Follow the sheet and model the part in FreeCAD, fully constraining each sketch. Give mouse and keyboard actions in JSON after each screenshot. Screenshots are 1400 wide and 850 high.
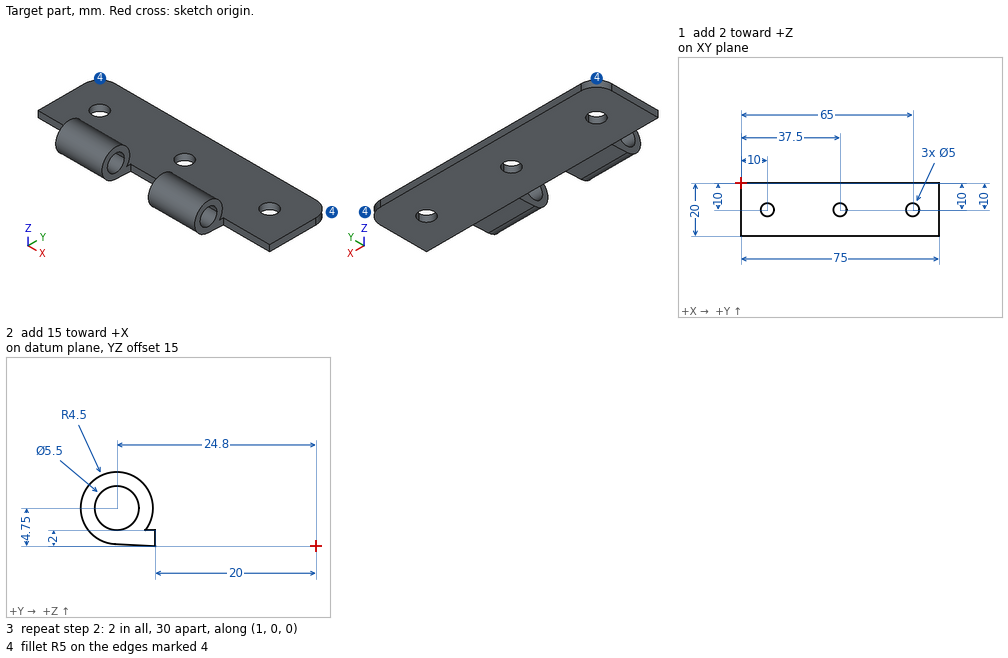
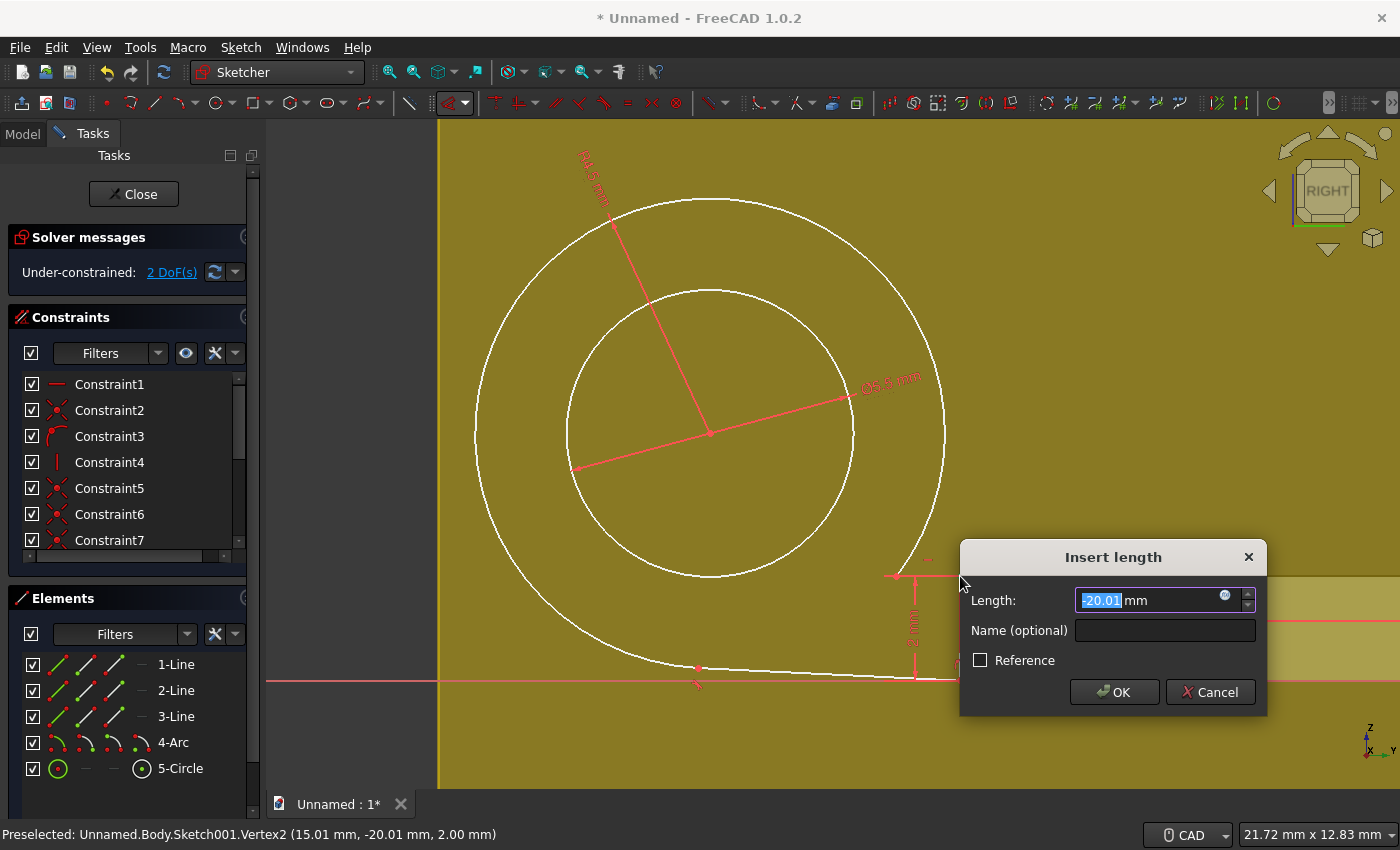
{"action": "type", "text": "-20"}
{"action": "key", "text": "Return"}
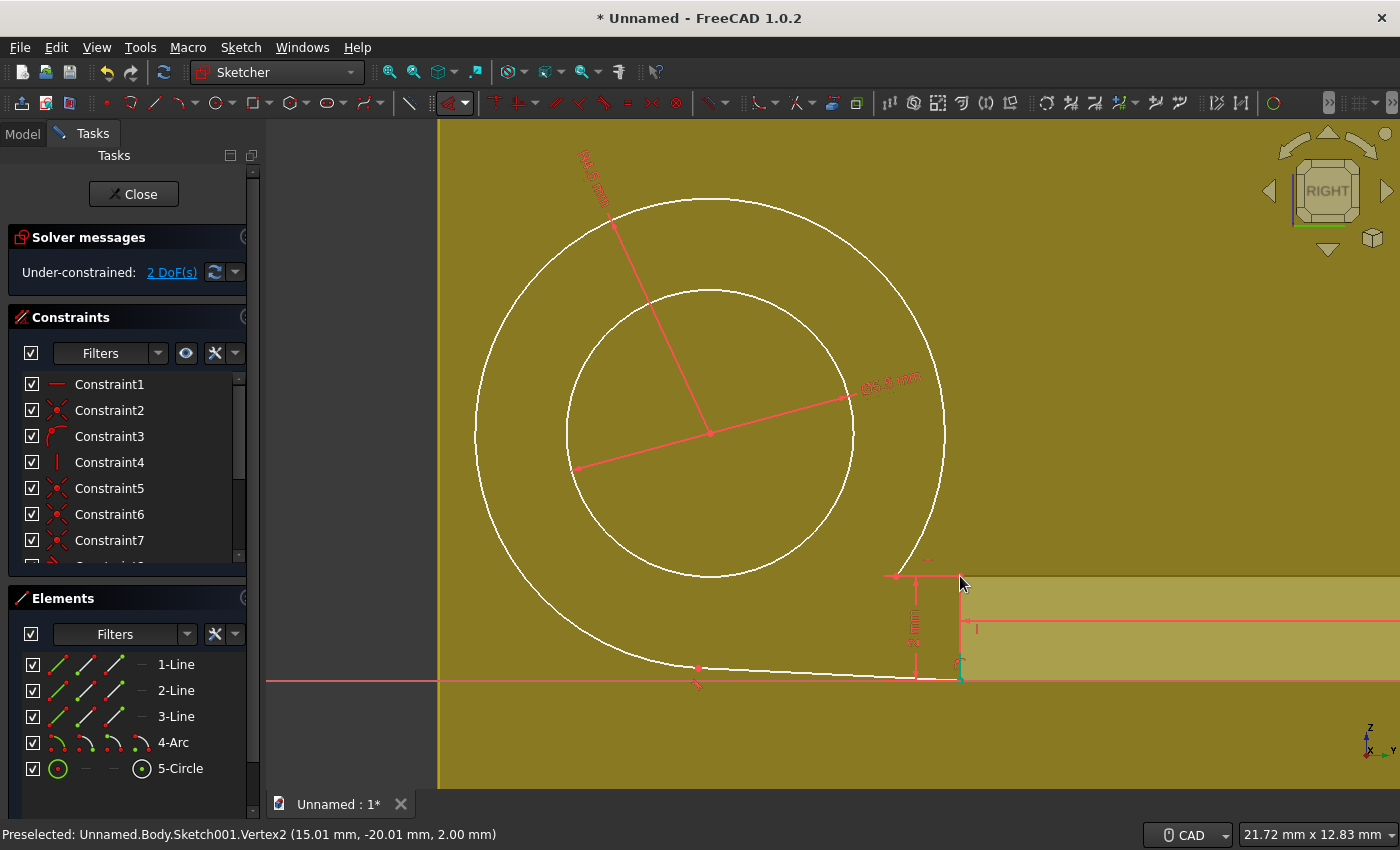
{"action": "left_click", "coordinate": [710, 433]}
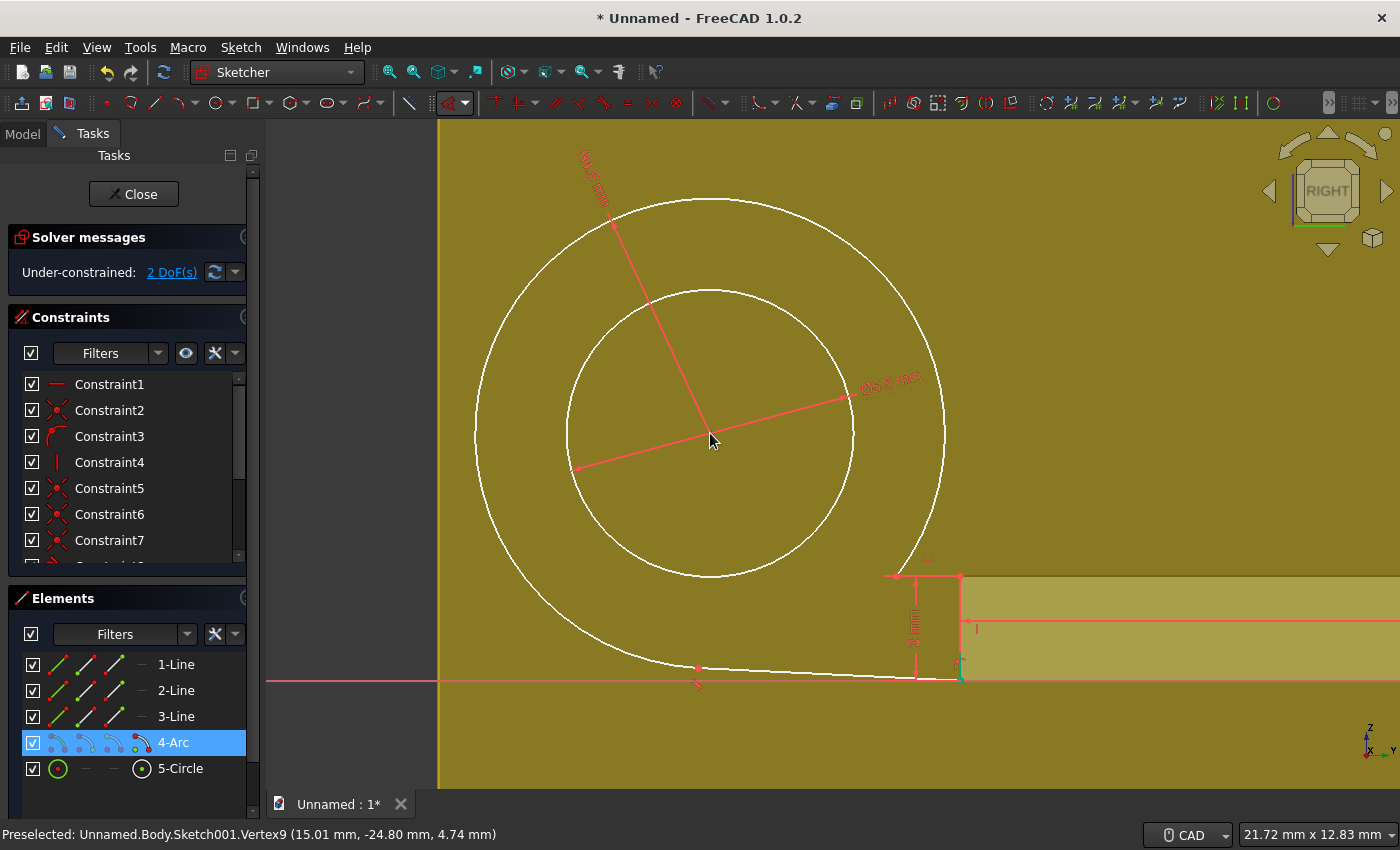
{"action": "key", "text": "l"}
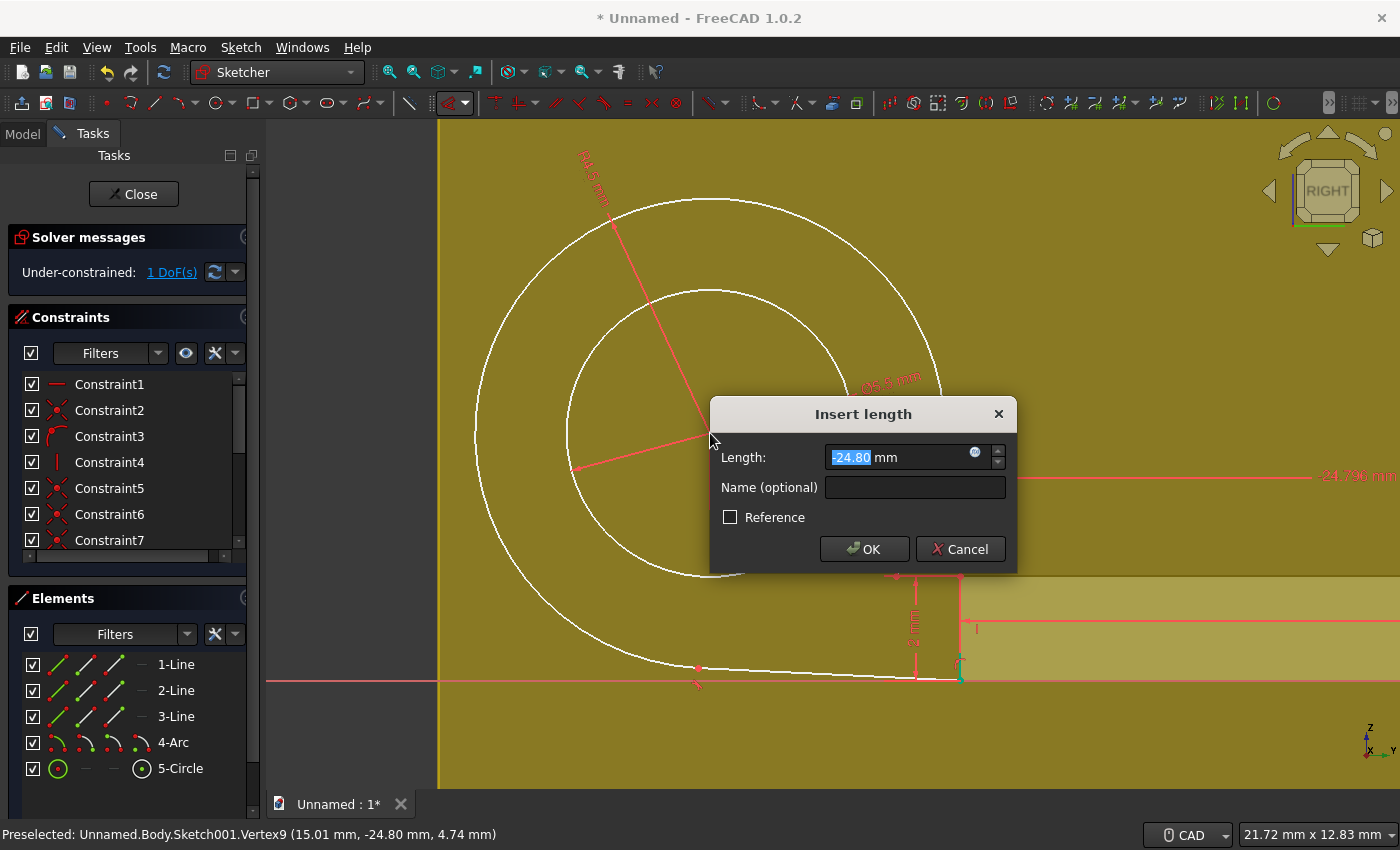
{"action": "type", "text": "-24.8"}
{"action": "key", "text": "Return"}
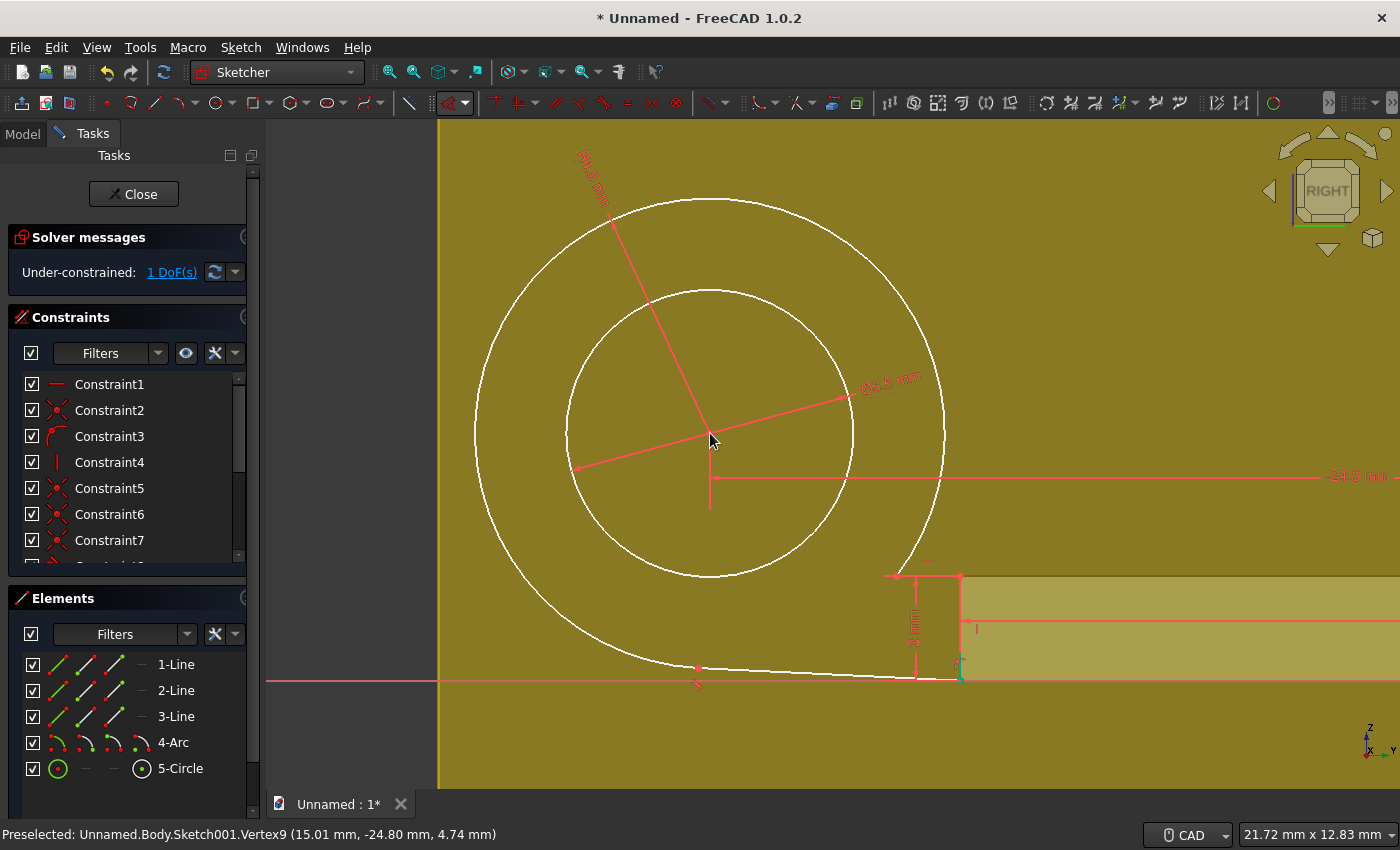
{"action": "left_click", "coordinate": [710, 433]}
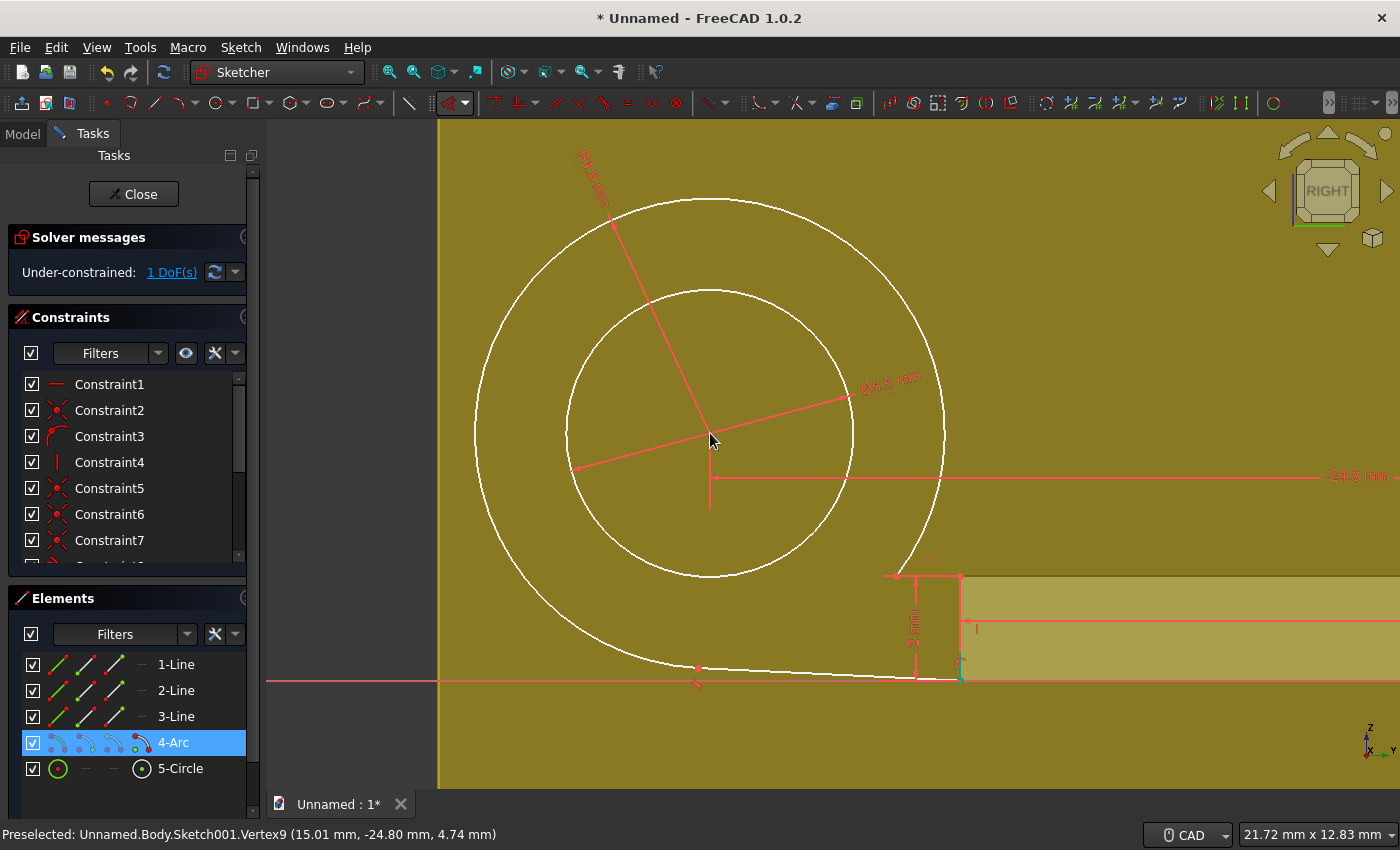
{"action": "key", "text": "i"}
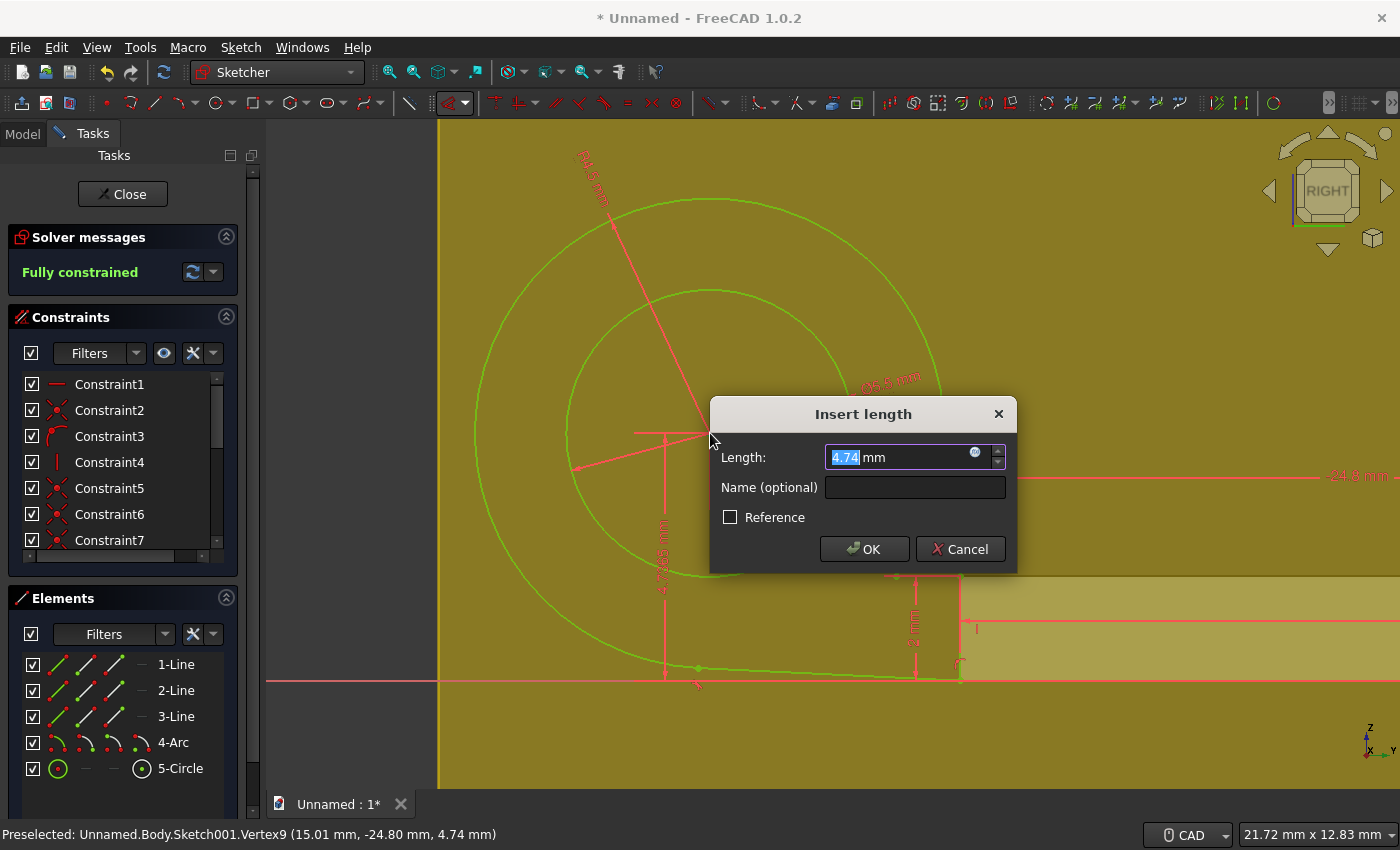
{"action": "type", "text": "4.75"}
{"action": "key", "text": "Return"}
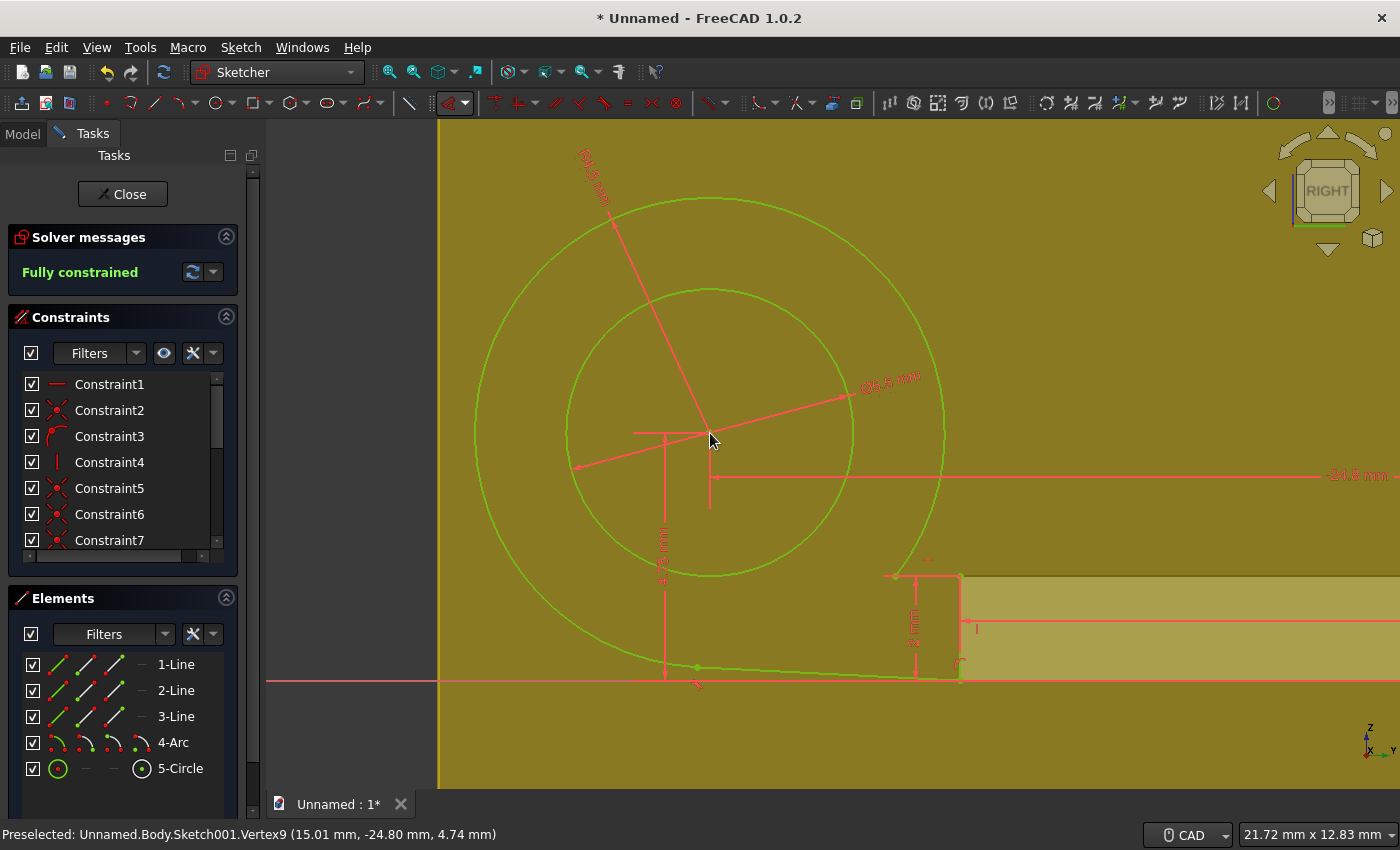
{"action": "left_click", "coordinate": [123, 194]}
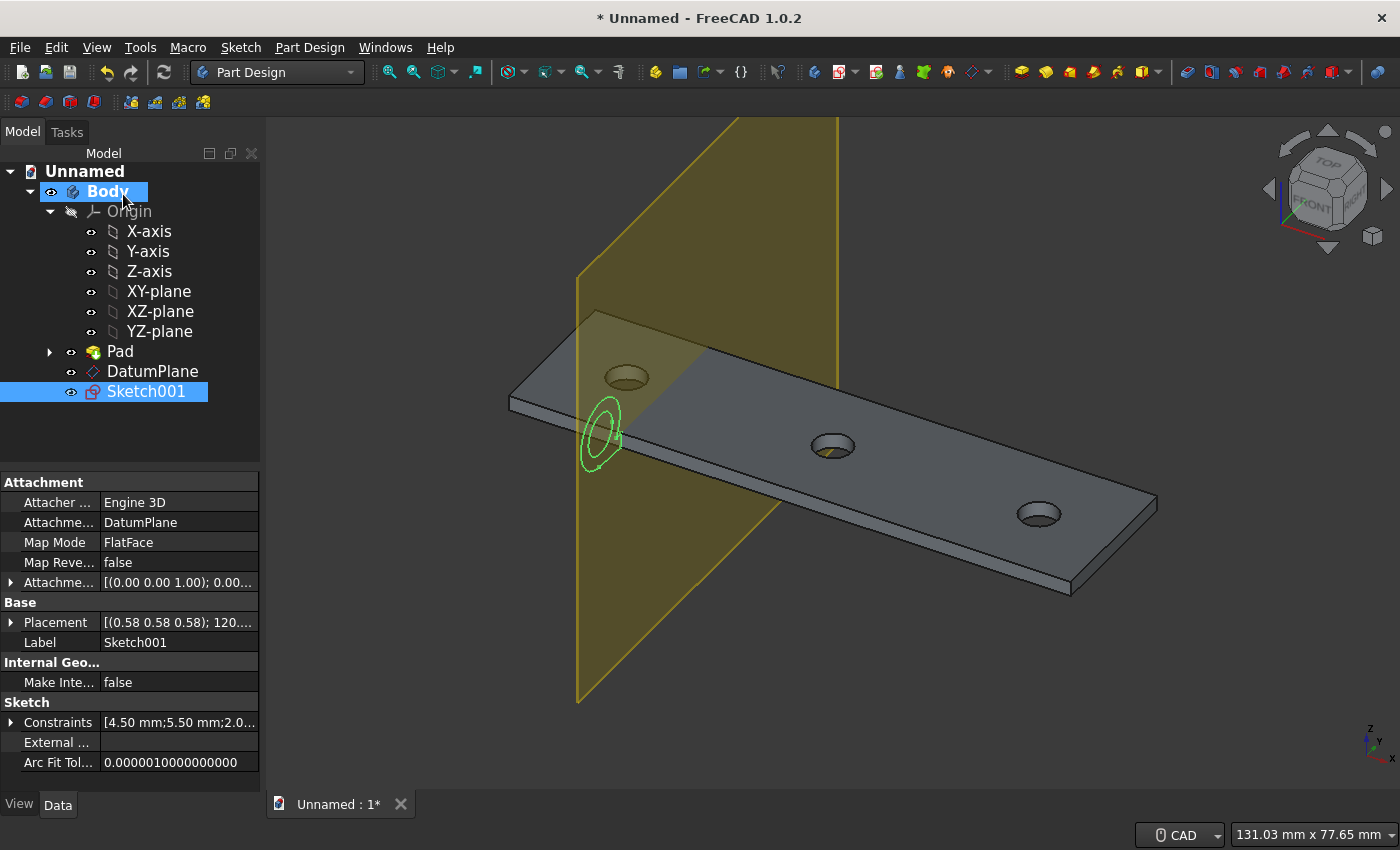
{"action": "left_click", "coordinate": [1022, 72]}